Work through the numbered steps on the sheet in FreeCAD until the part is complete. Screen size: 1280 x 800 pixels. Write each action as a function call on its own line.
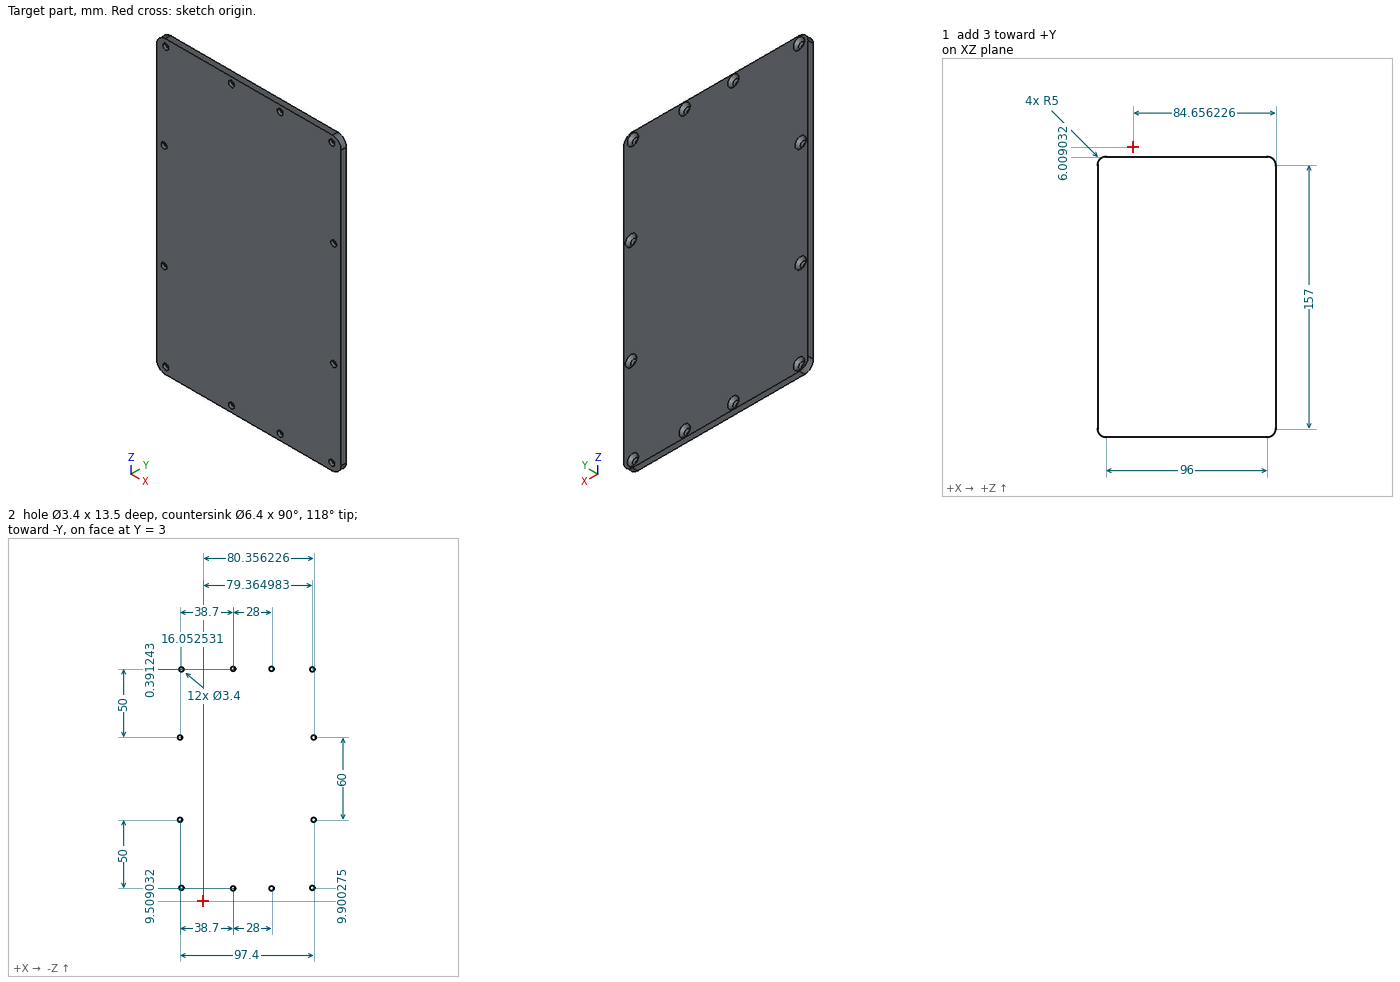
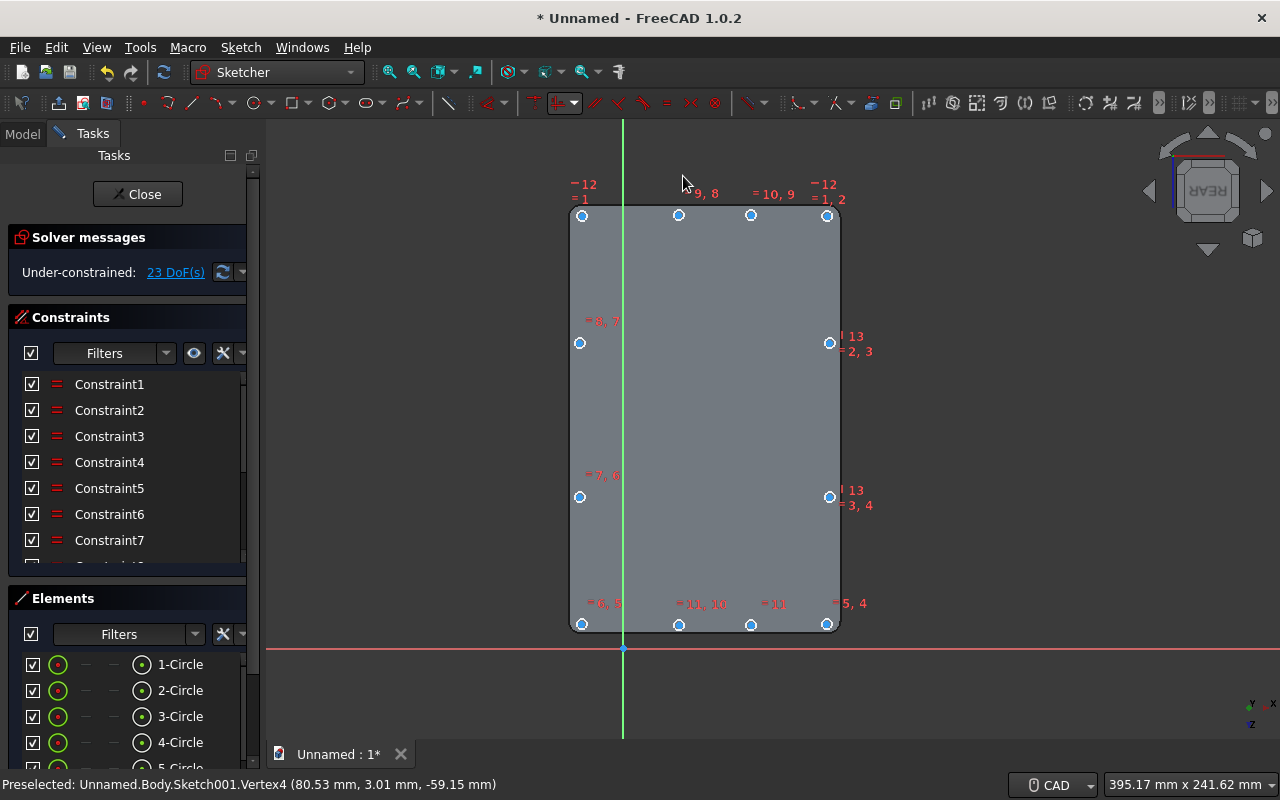
click(827, 216)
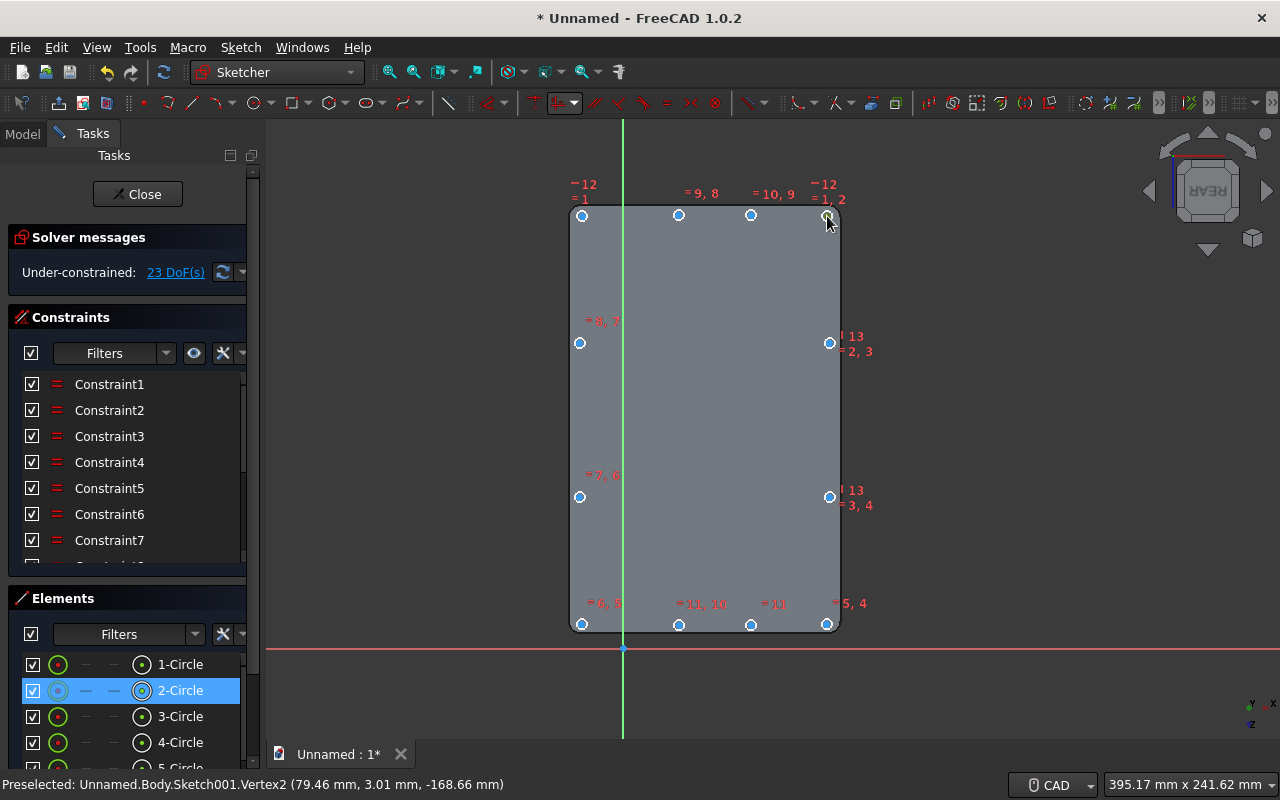
click(827, 624)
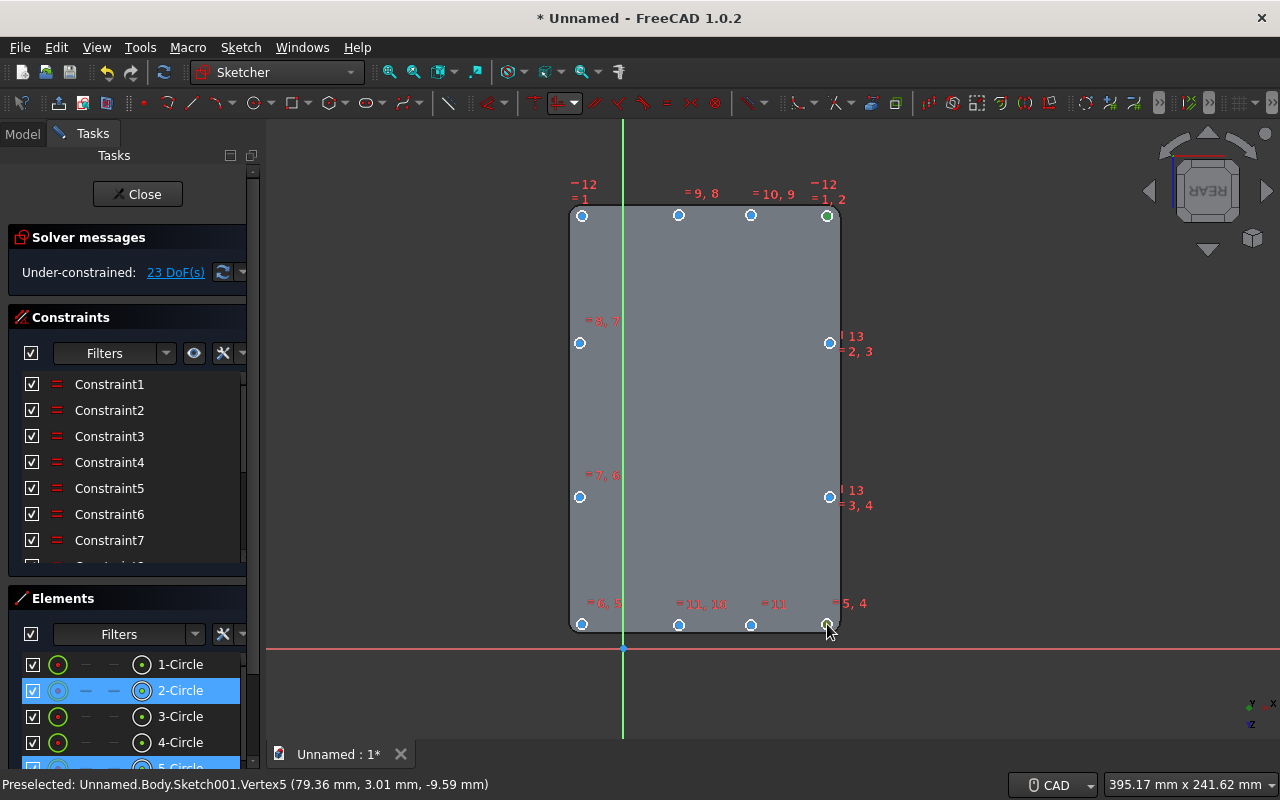
click(576, 104)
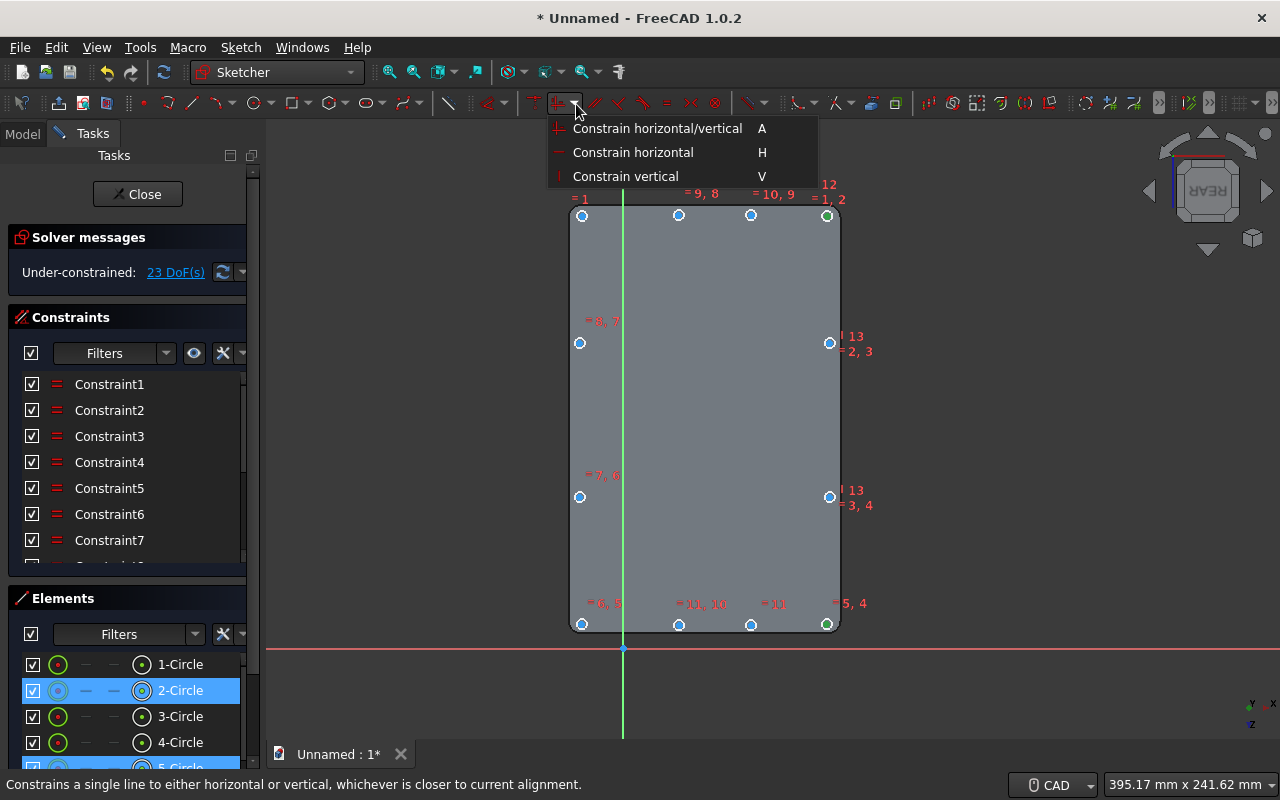
click(683, 176)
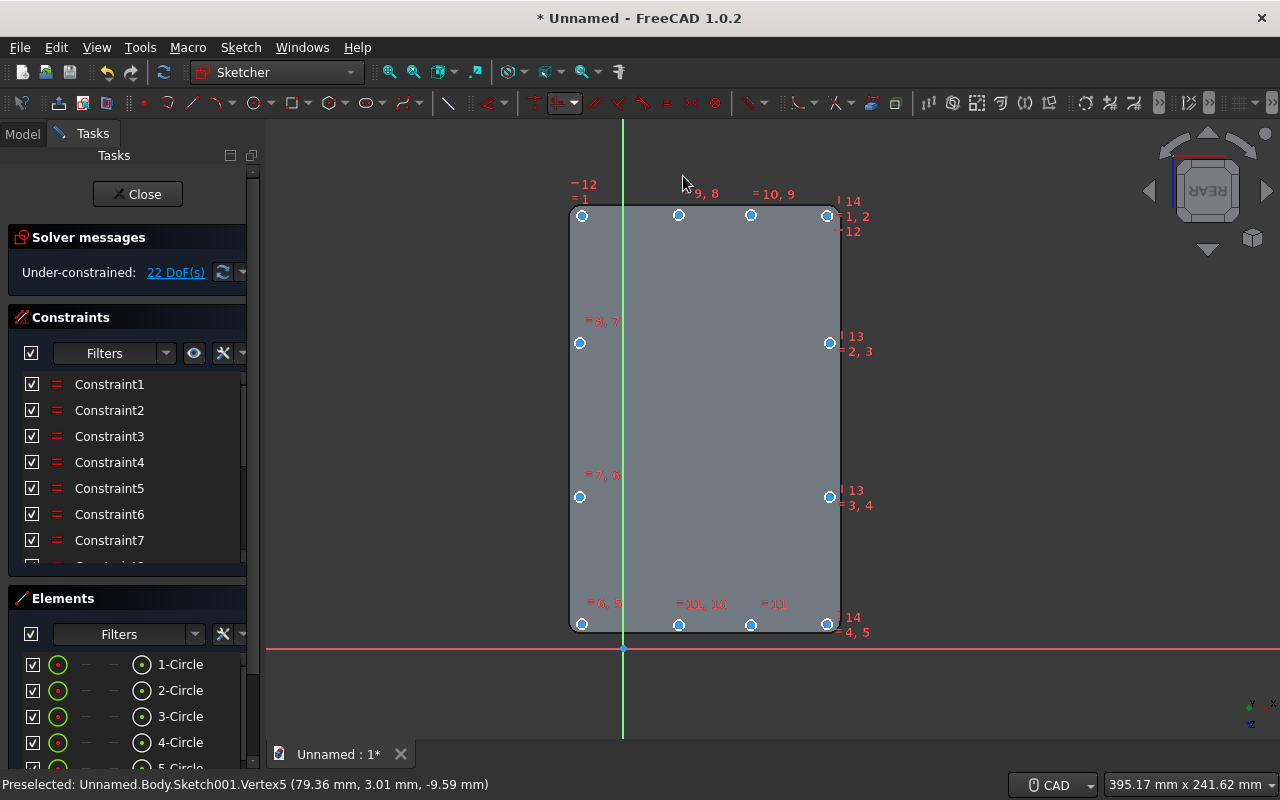
click(582, 216)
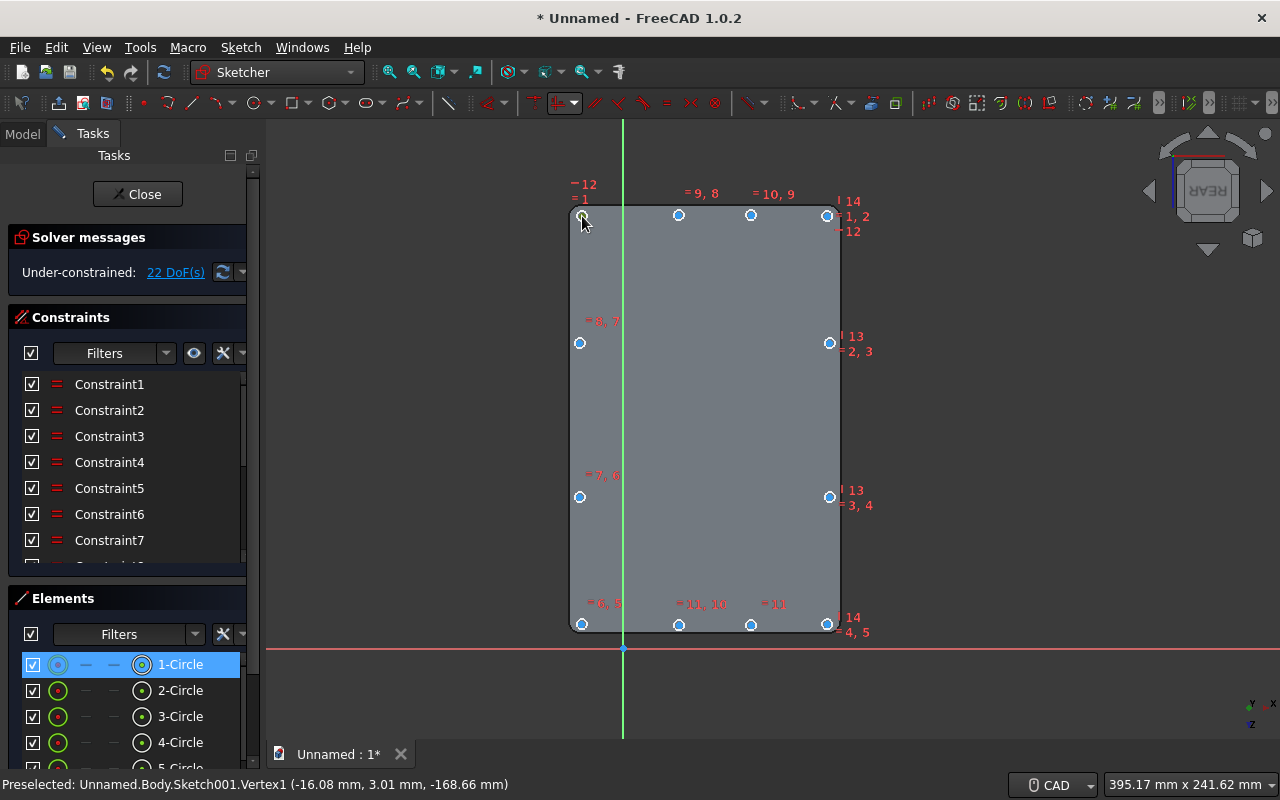
click(582, 624)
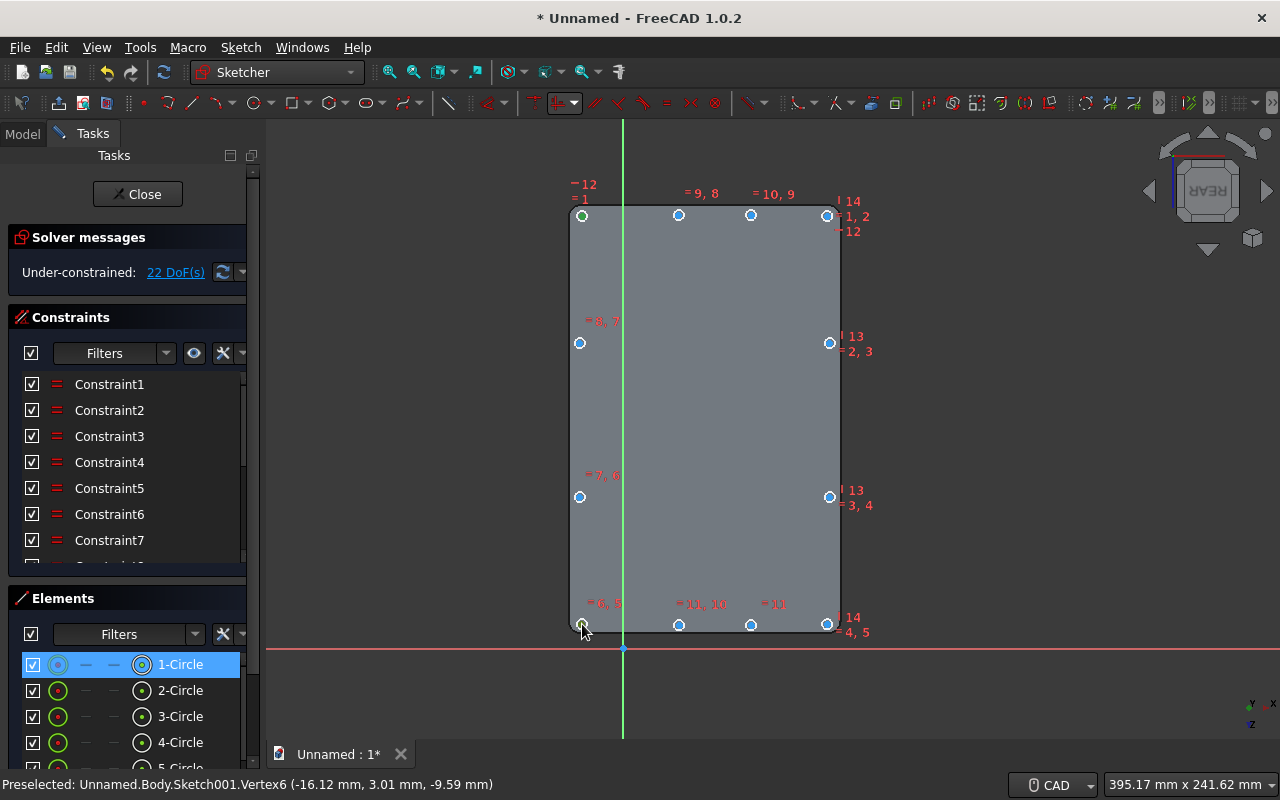
key(v)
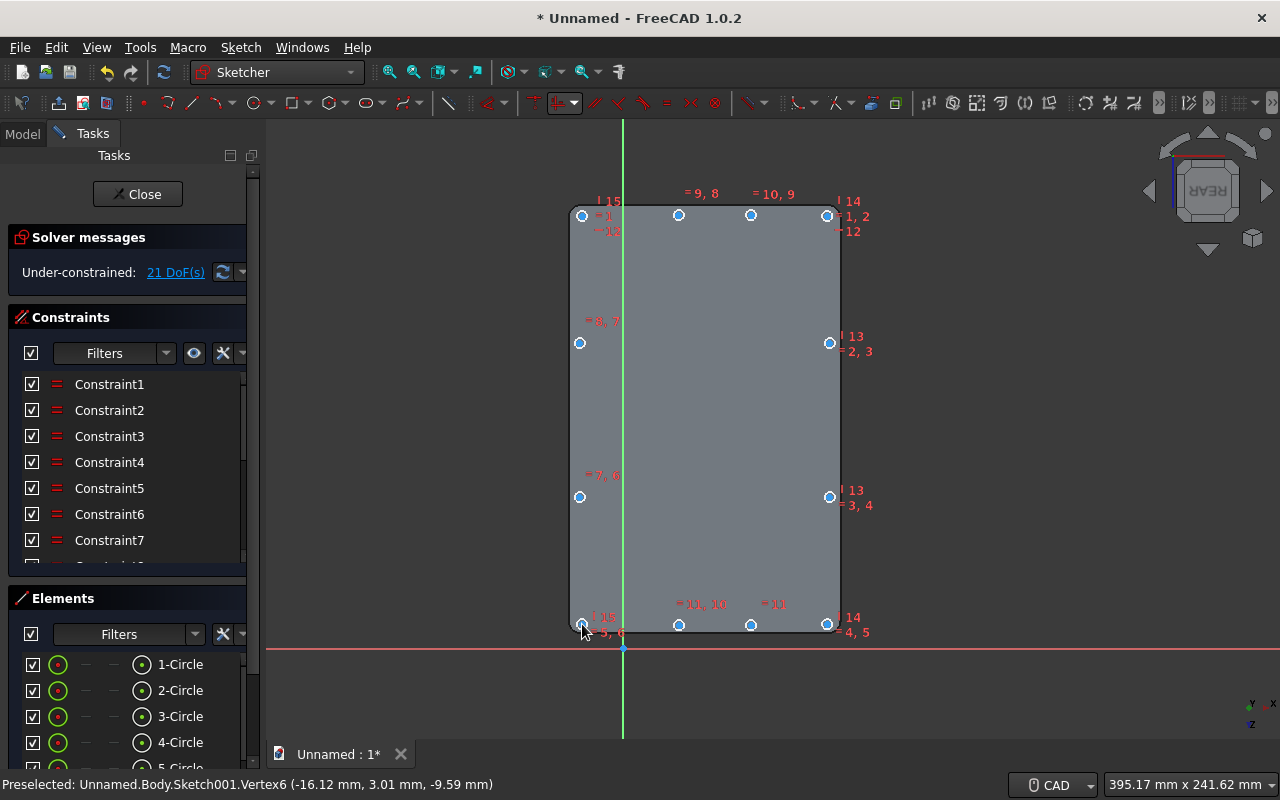
click(827, 624)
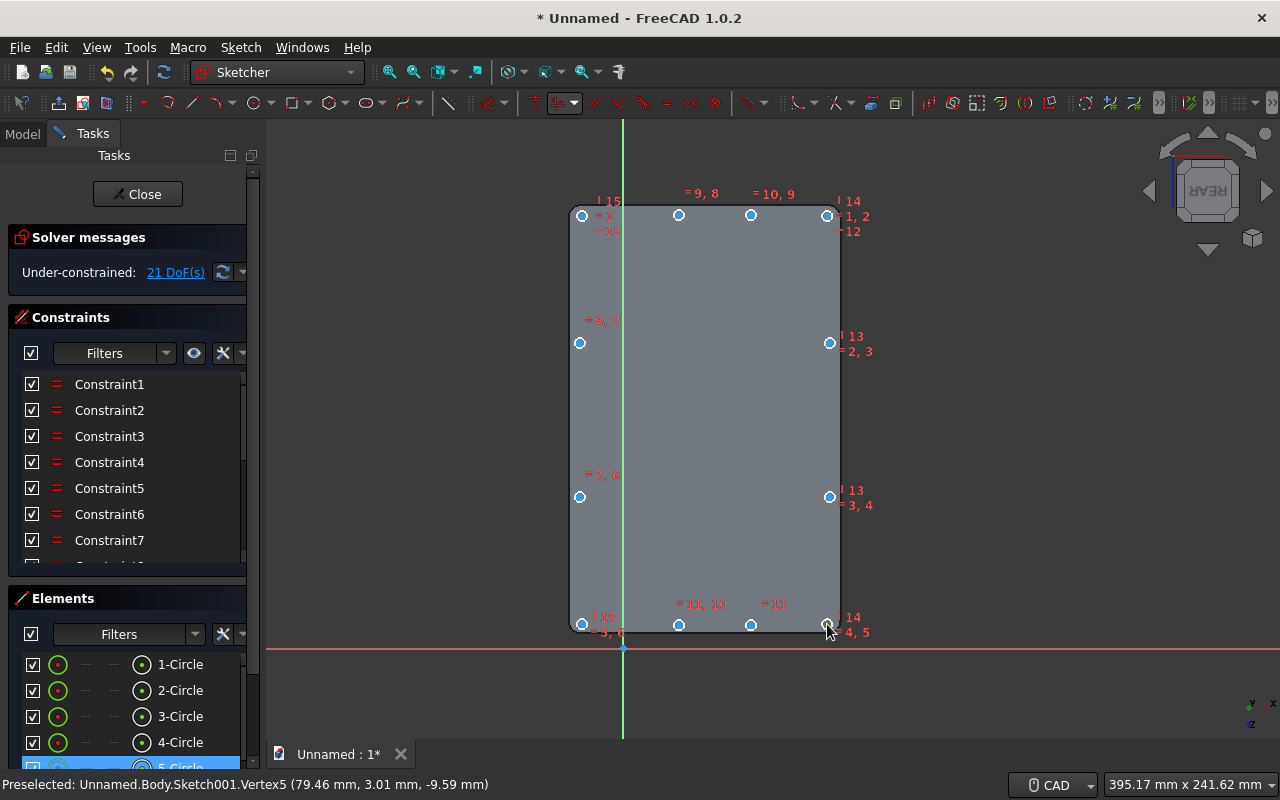
click(582, 624)